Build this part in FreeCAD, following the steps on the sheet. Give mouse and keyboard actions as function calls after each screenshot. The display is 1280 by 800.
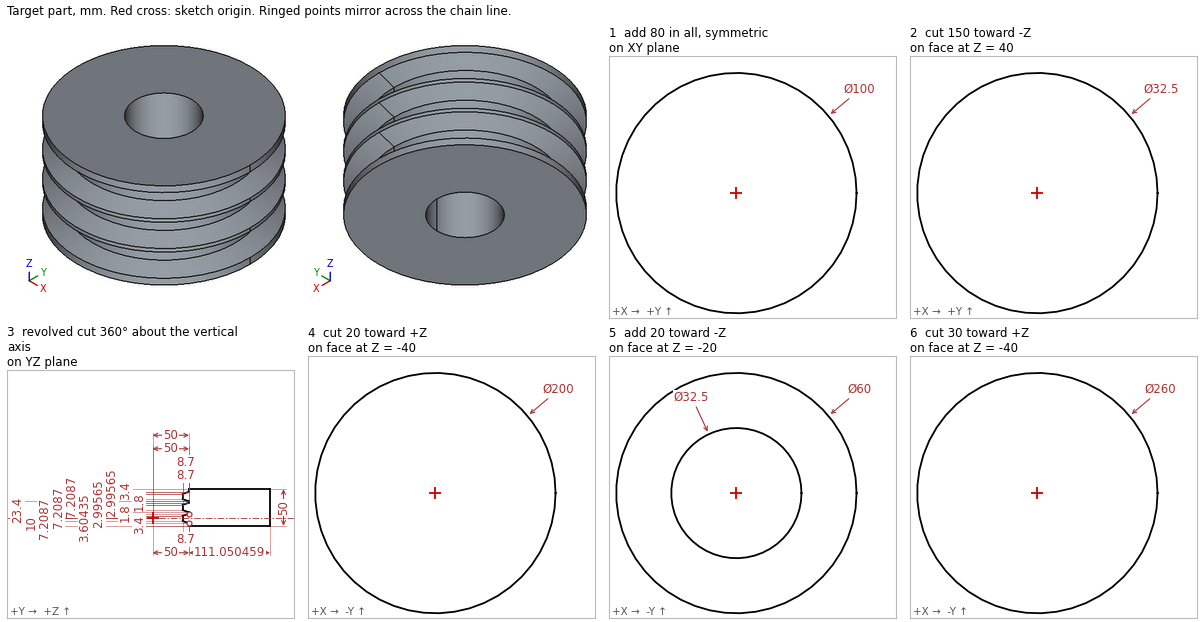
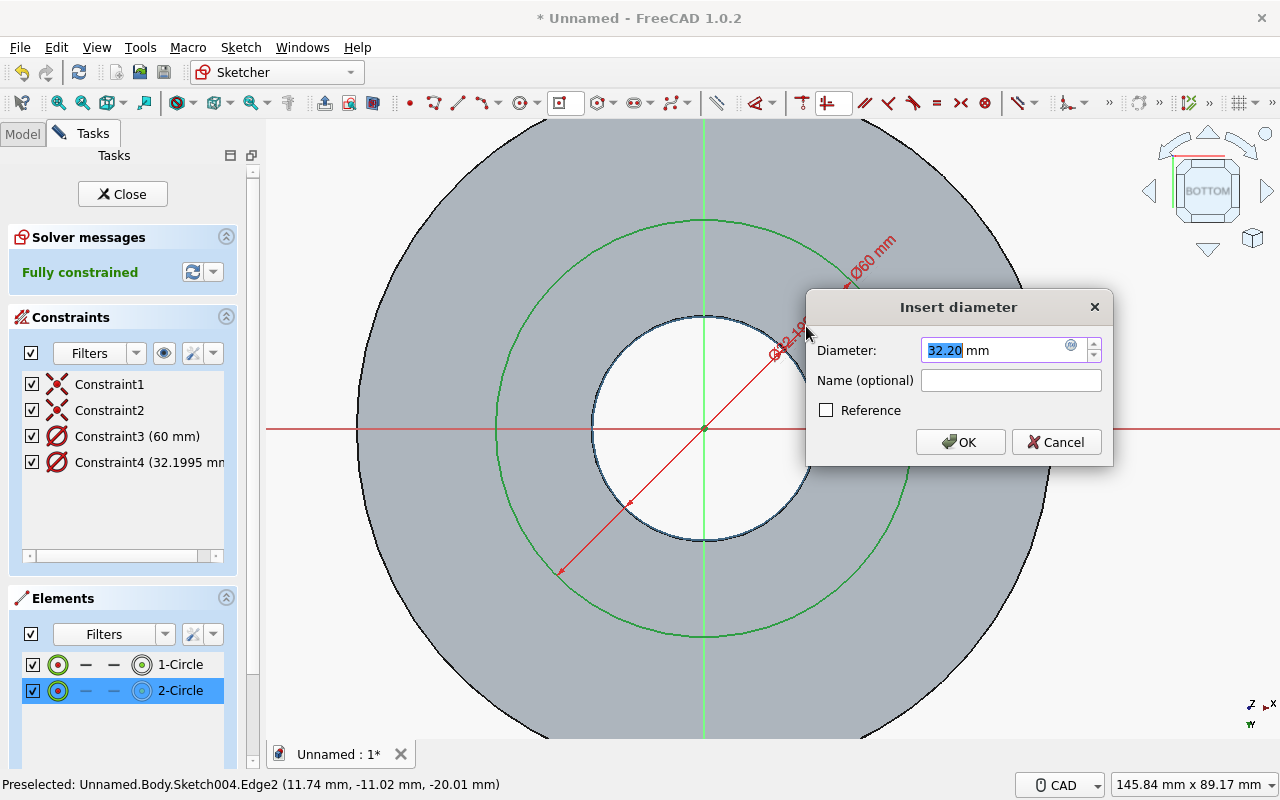
text(32.5)
key(Return)
key(Escape)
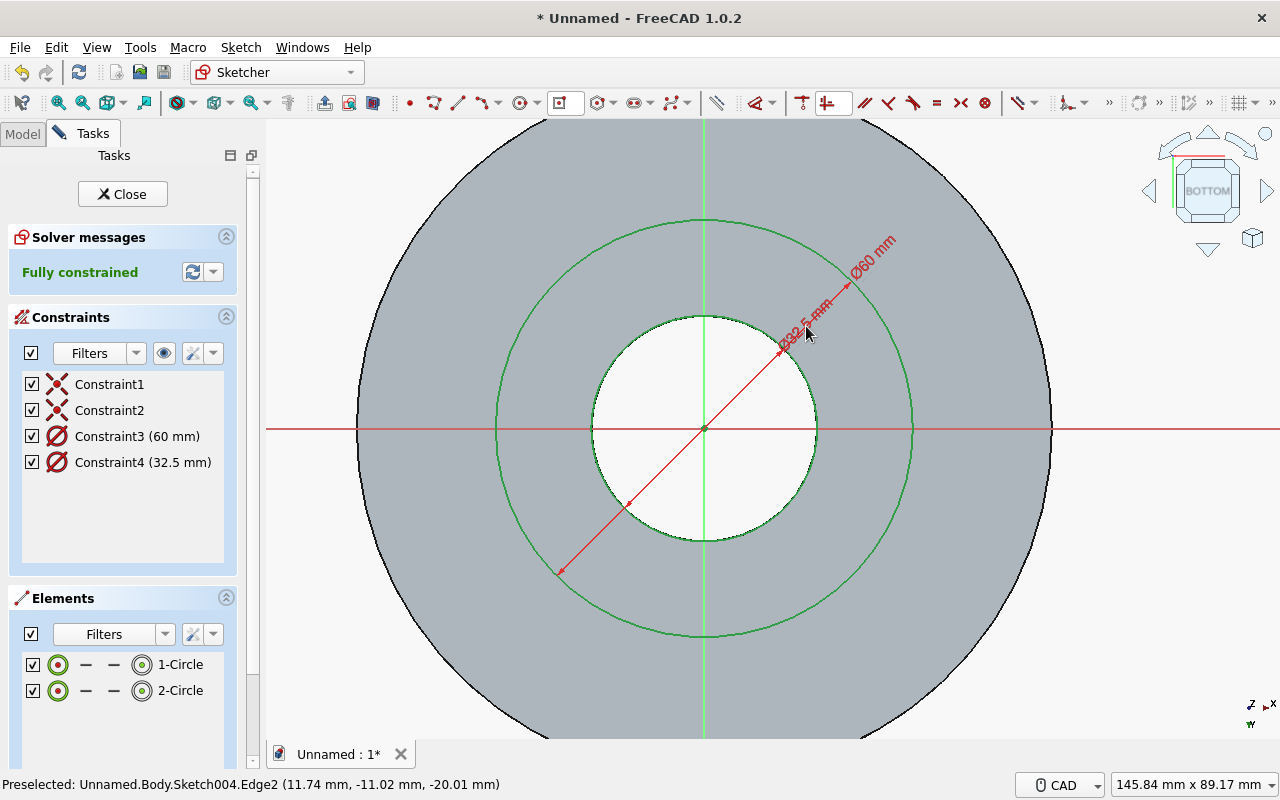
click(123, 194)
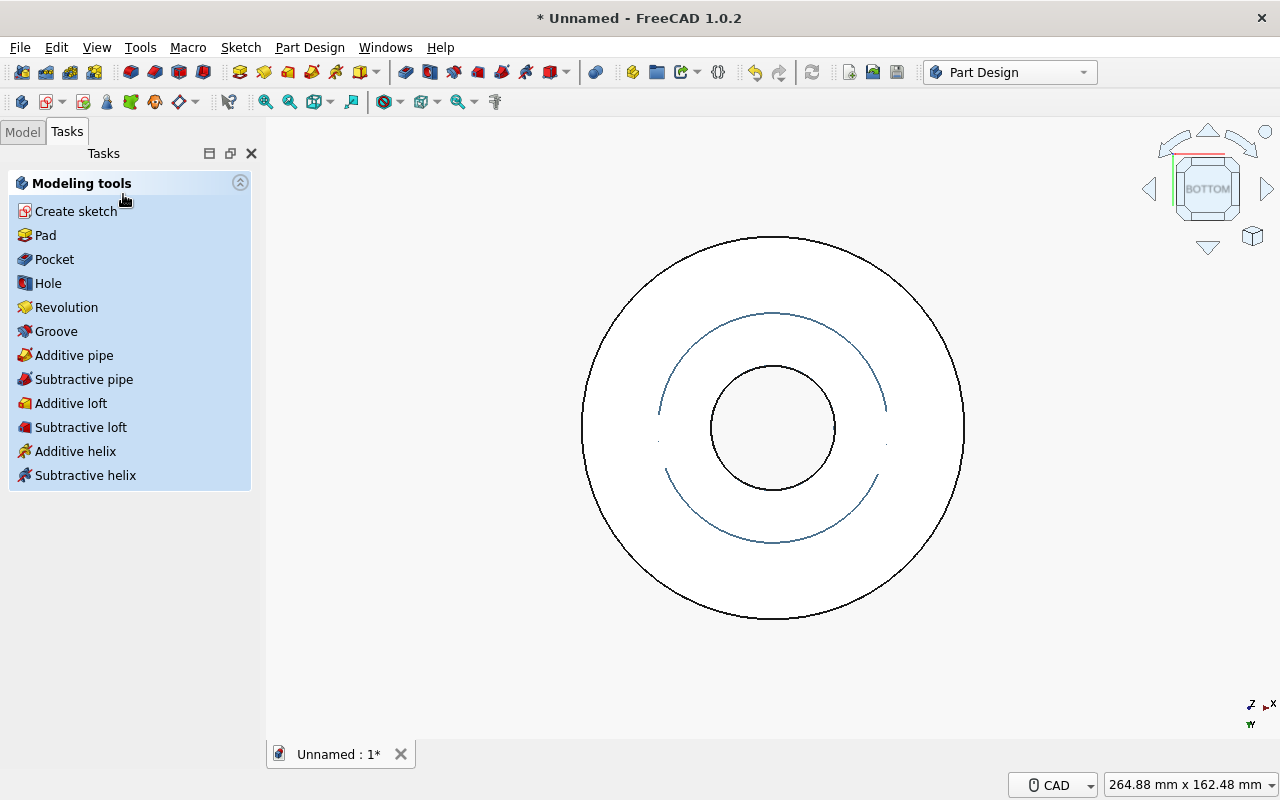
click(240, 72)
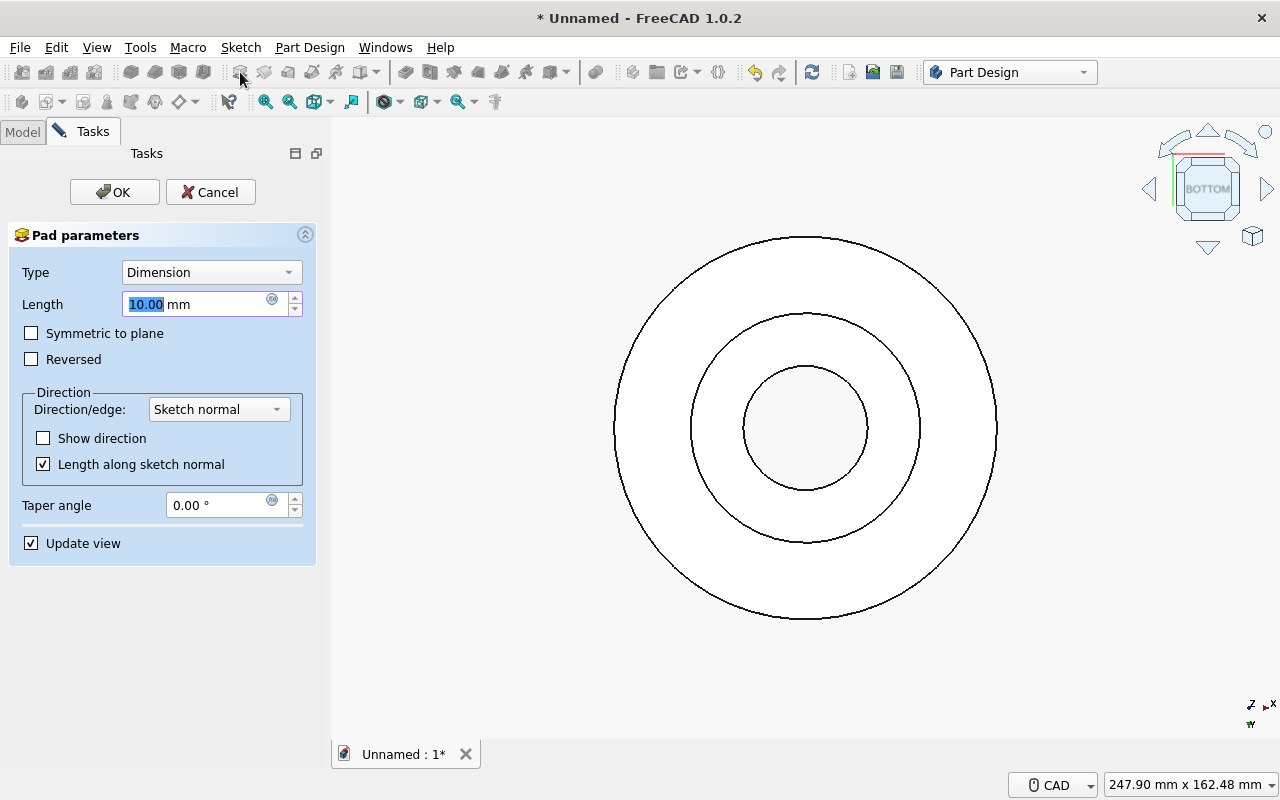
text(20)
key(Tab)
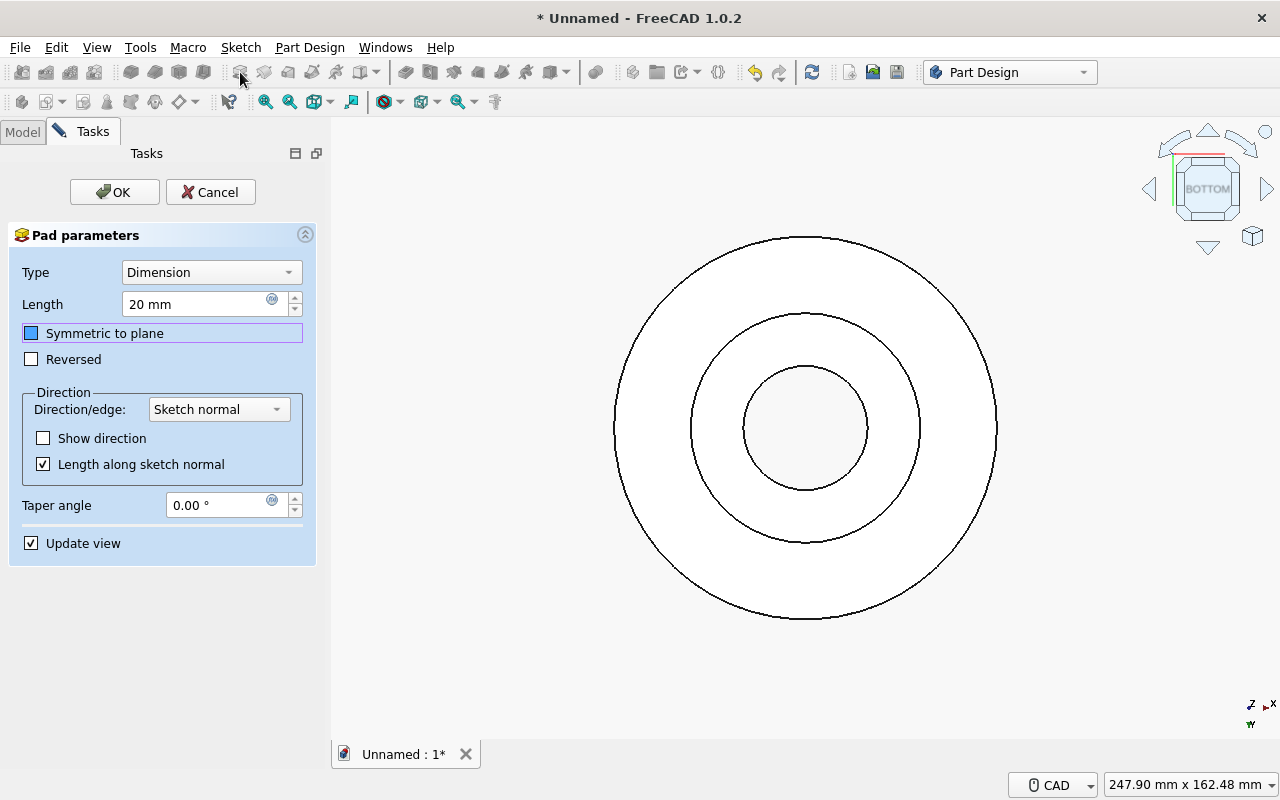
click(115, 192)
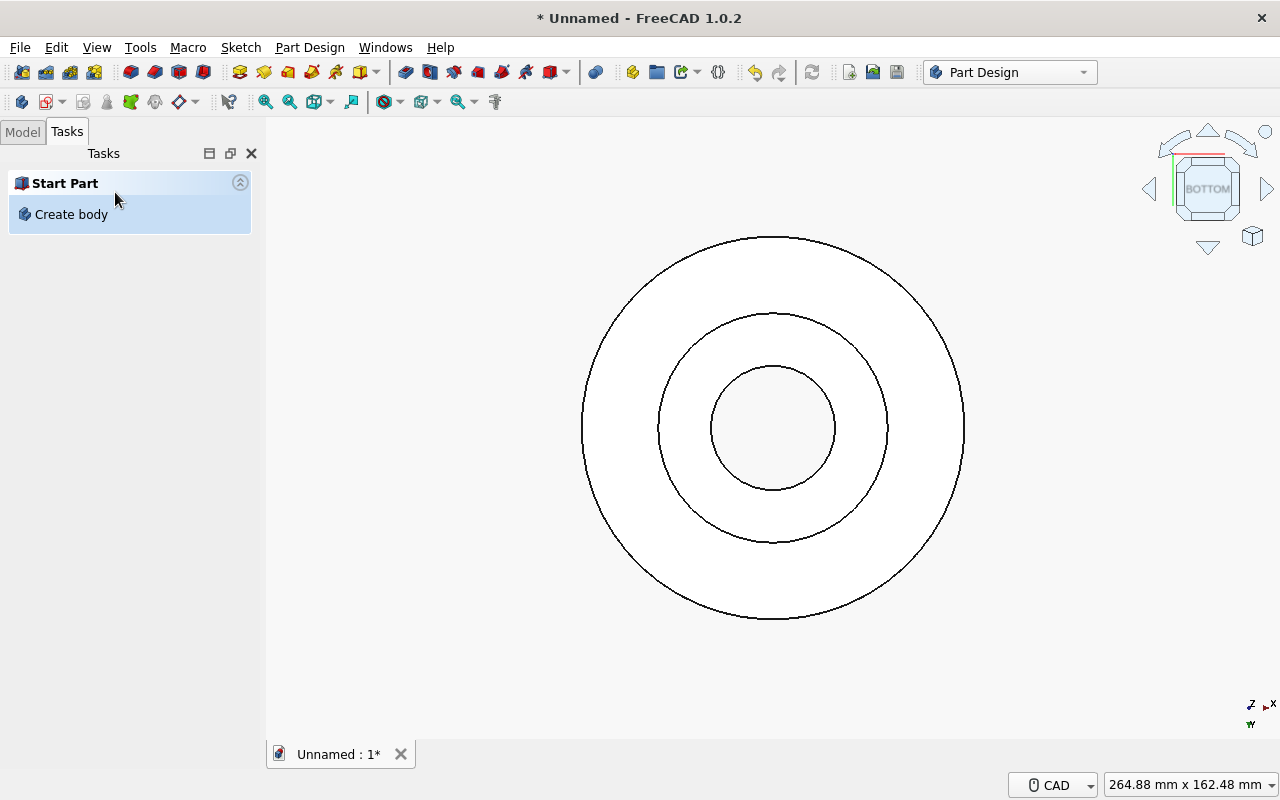
click(707, 493)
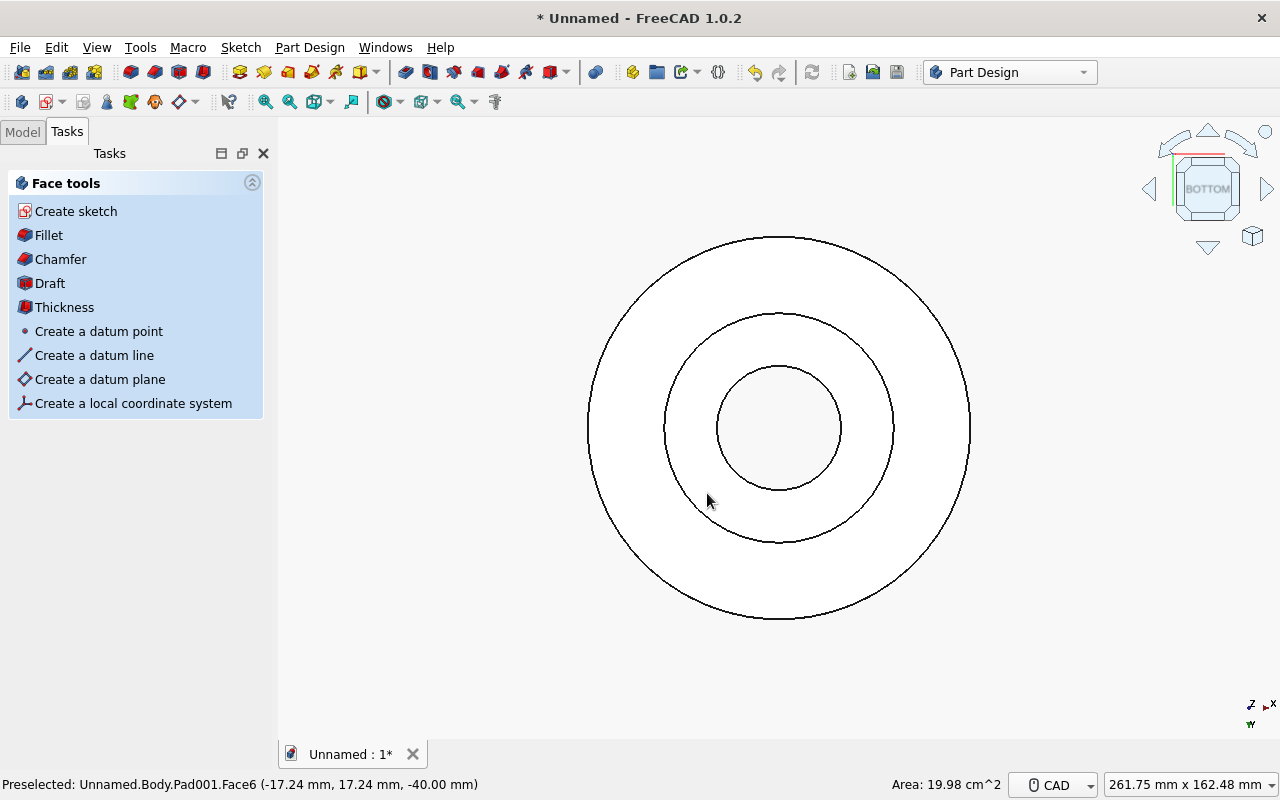
click(46, 102)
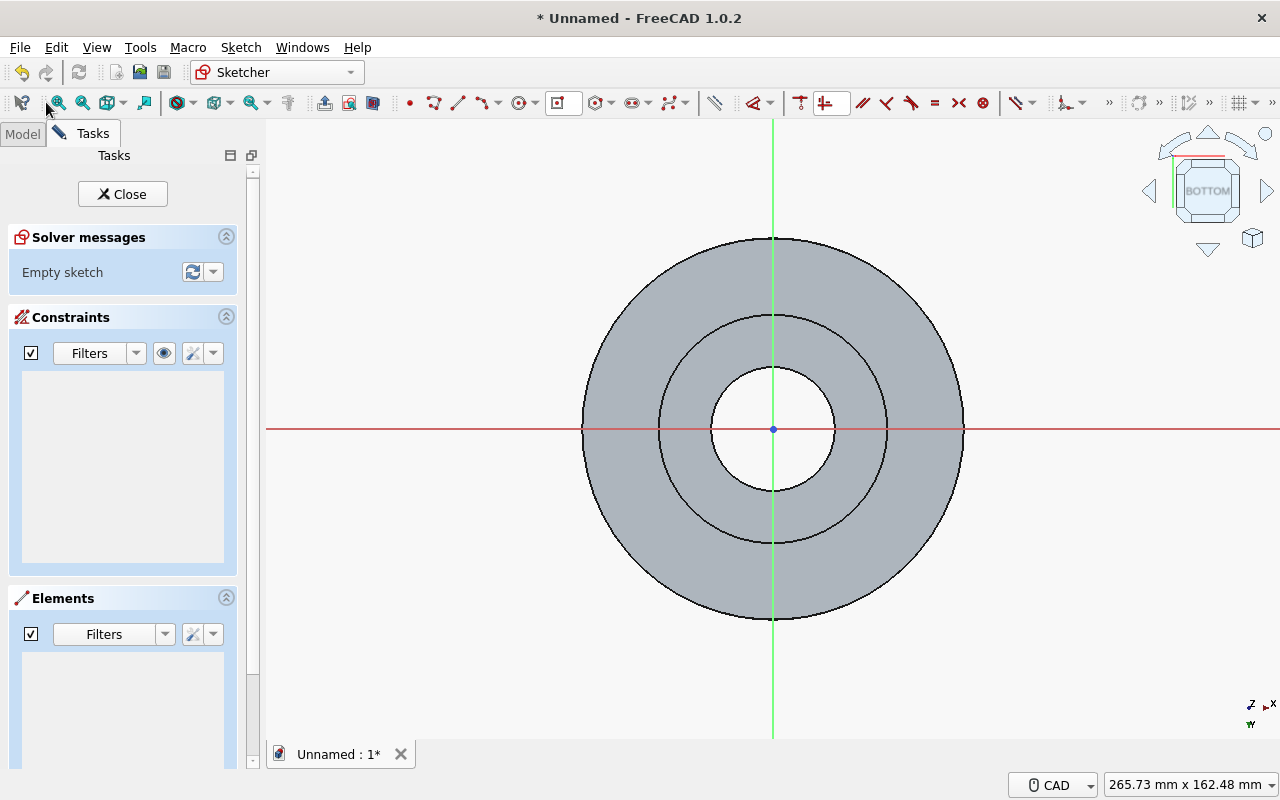
scroll(665, 429, down, 5)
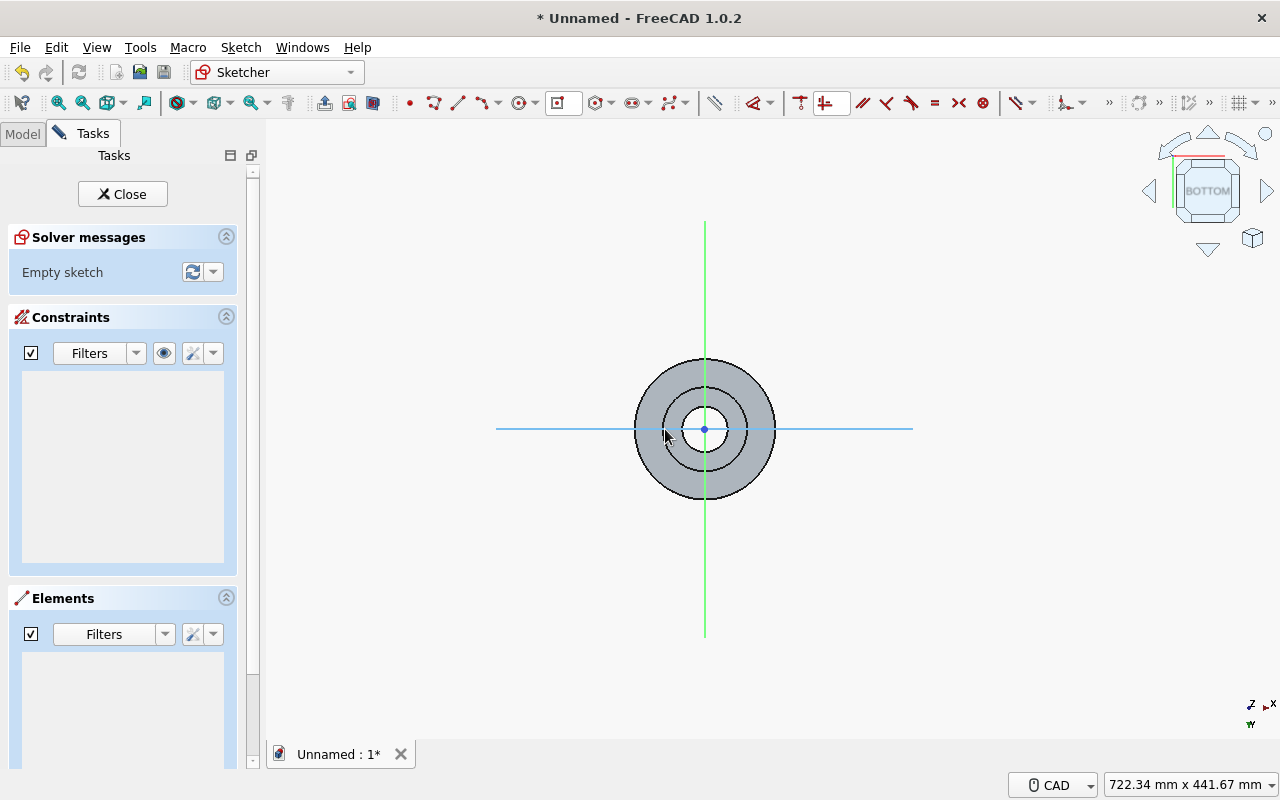
key(g)
key(c)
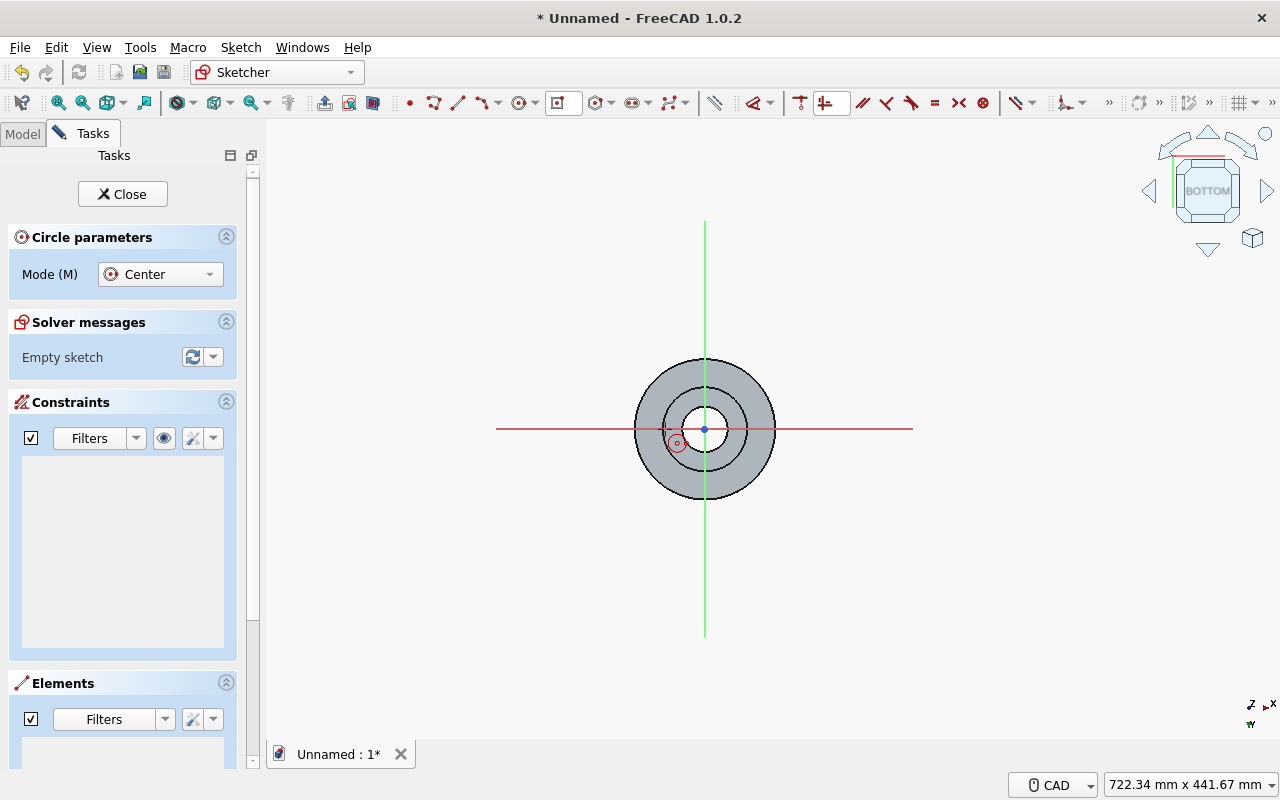
click(705, 429)
click(834, 300)
key(Escape)